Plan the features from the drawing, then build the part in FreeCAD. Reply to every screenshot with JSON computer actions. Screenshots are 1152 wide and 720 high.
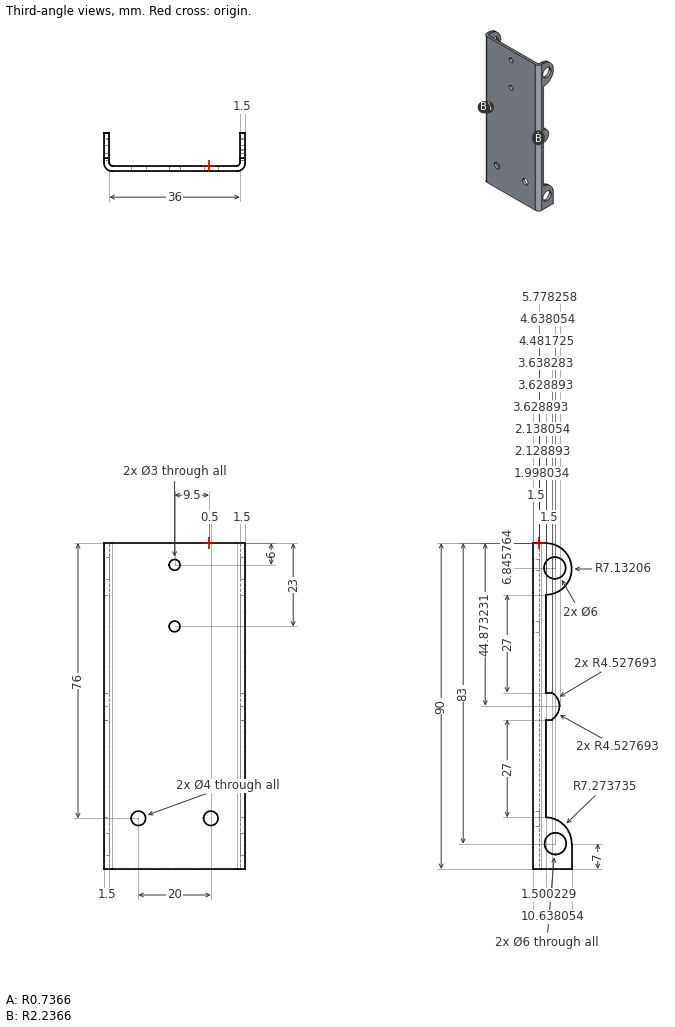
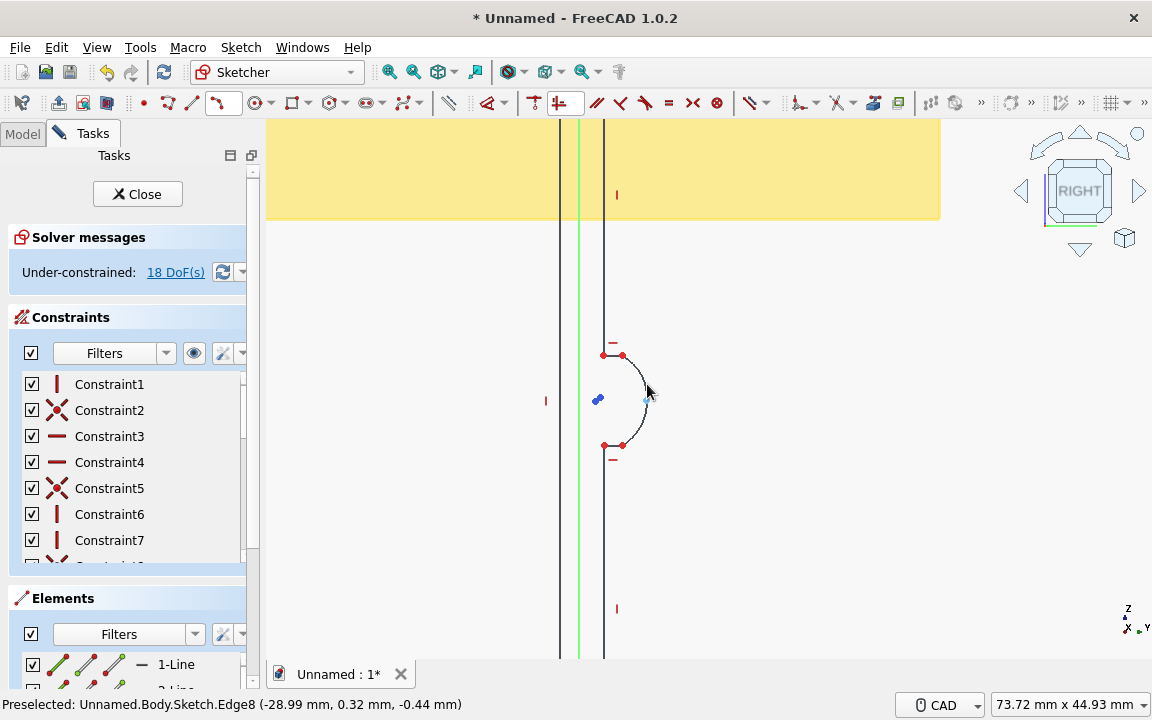
{"action": "left_click", "coordinate": [645, 384]}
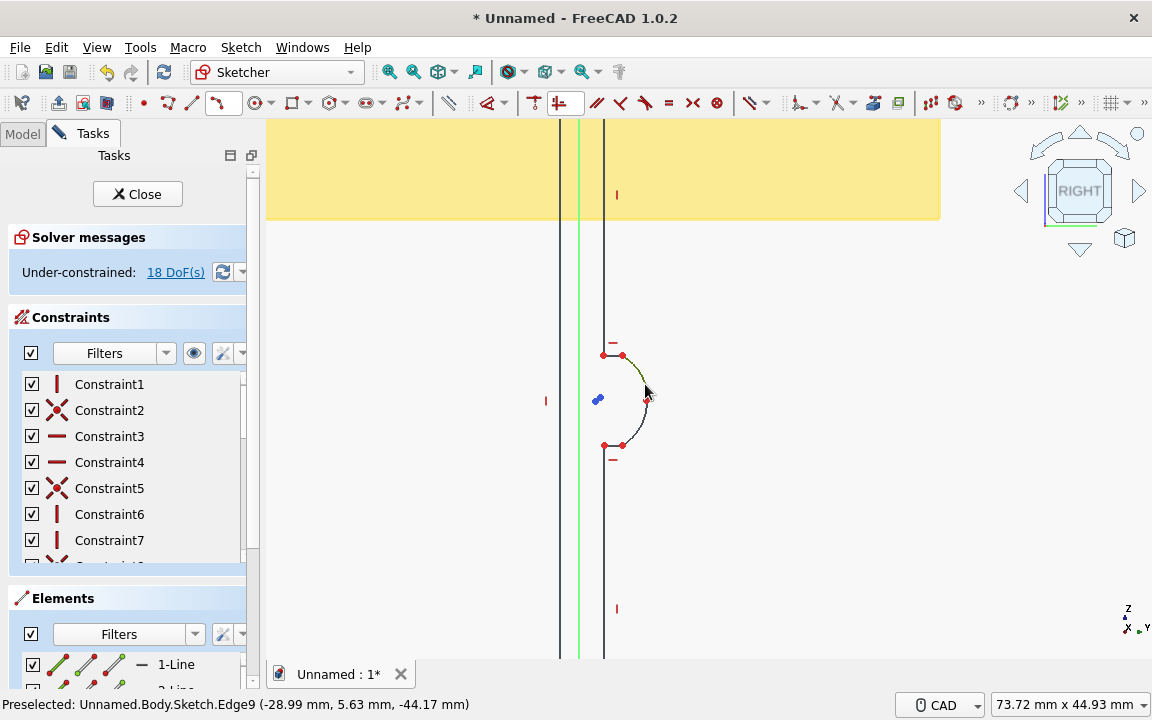
{"action": "left_click", "coordinate": [634, 435]}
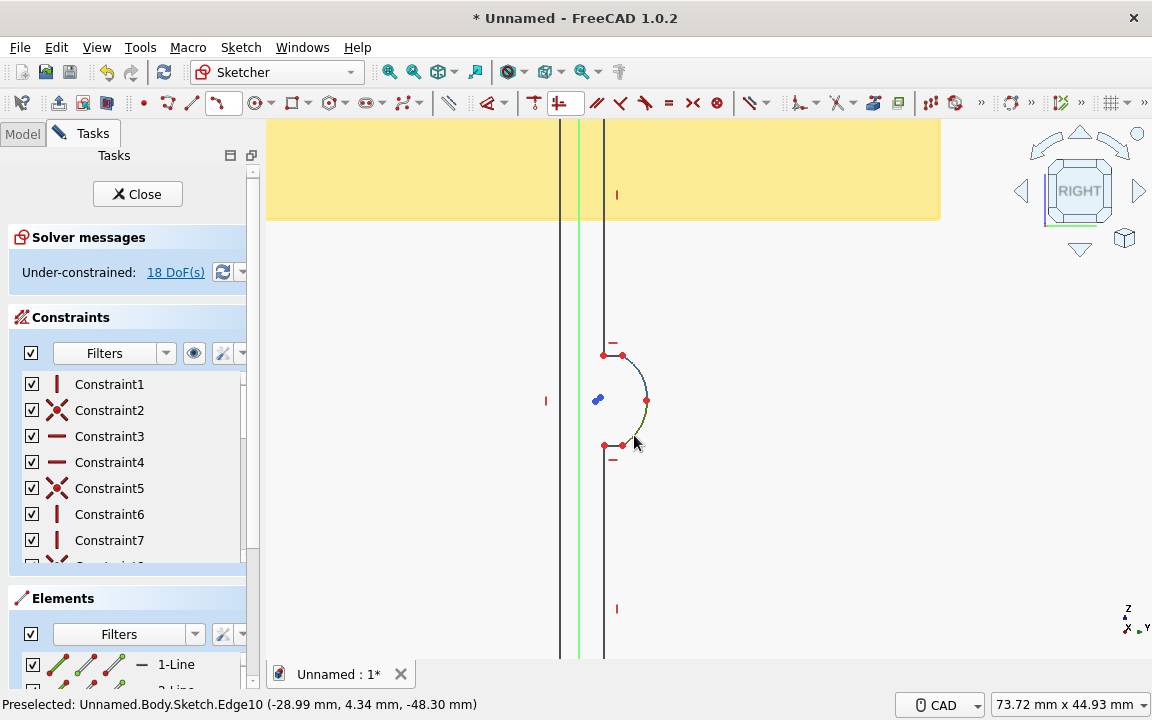
{"action": "key", "text": "e"}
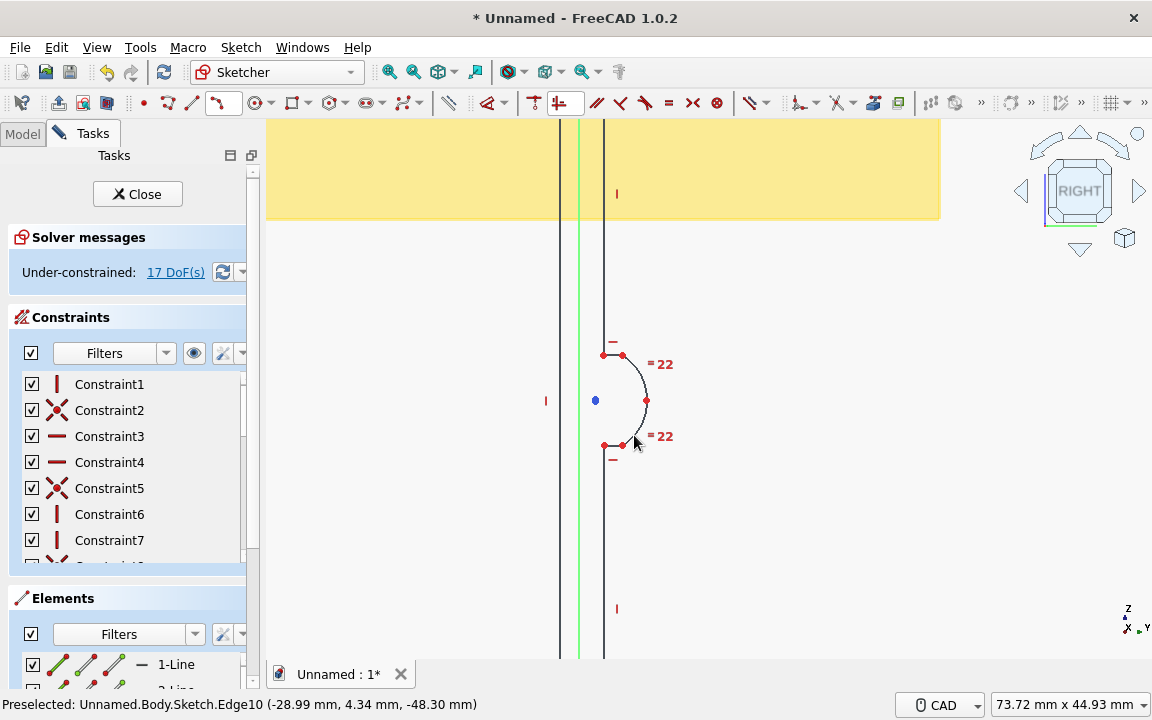
{"action": "left_click", "coordinate": [488, 104]}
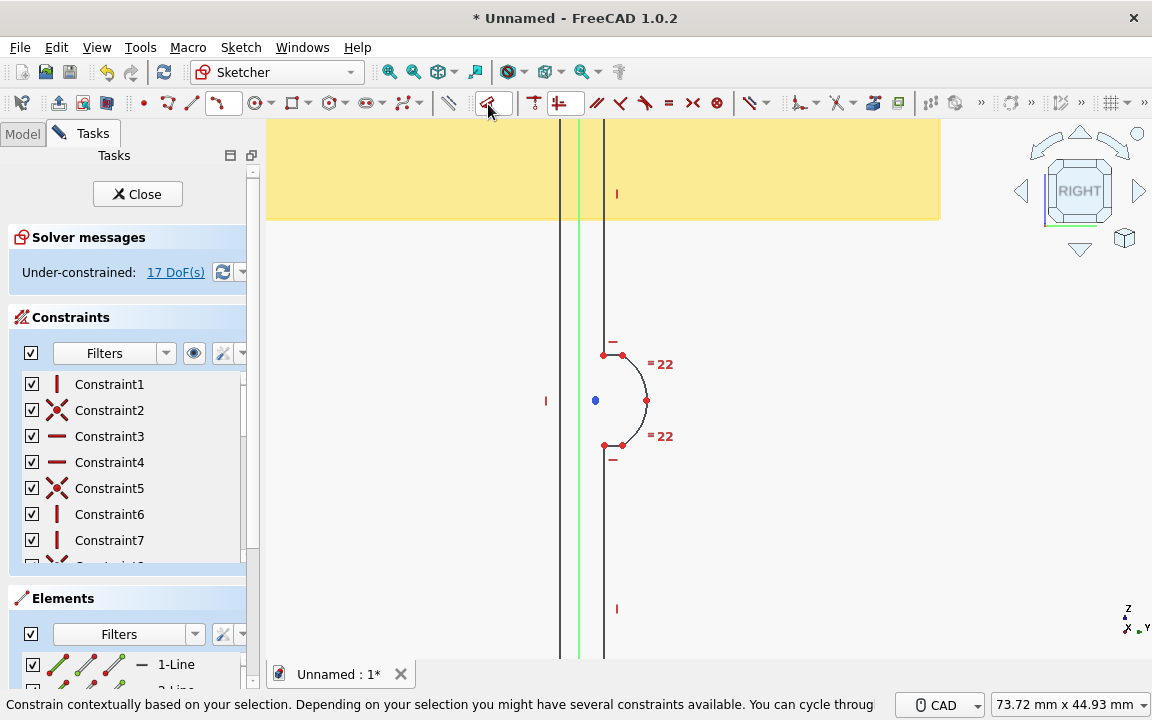
{"action": "left_click", "coordinate": [645, 385]}
{"action": "left_click", "coordinate": [676, 376]}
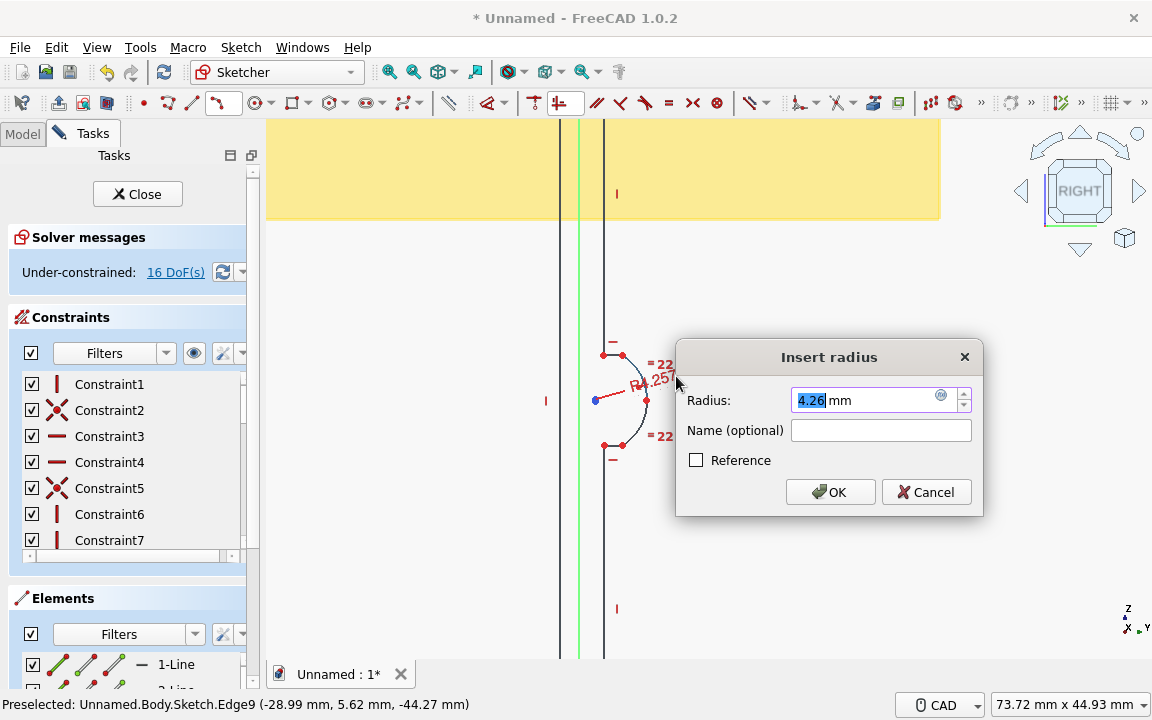
{"action": "type", "text": "4.527693"}
{"action": "key", "text": "Return"}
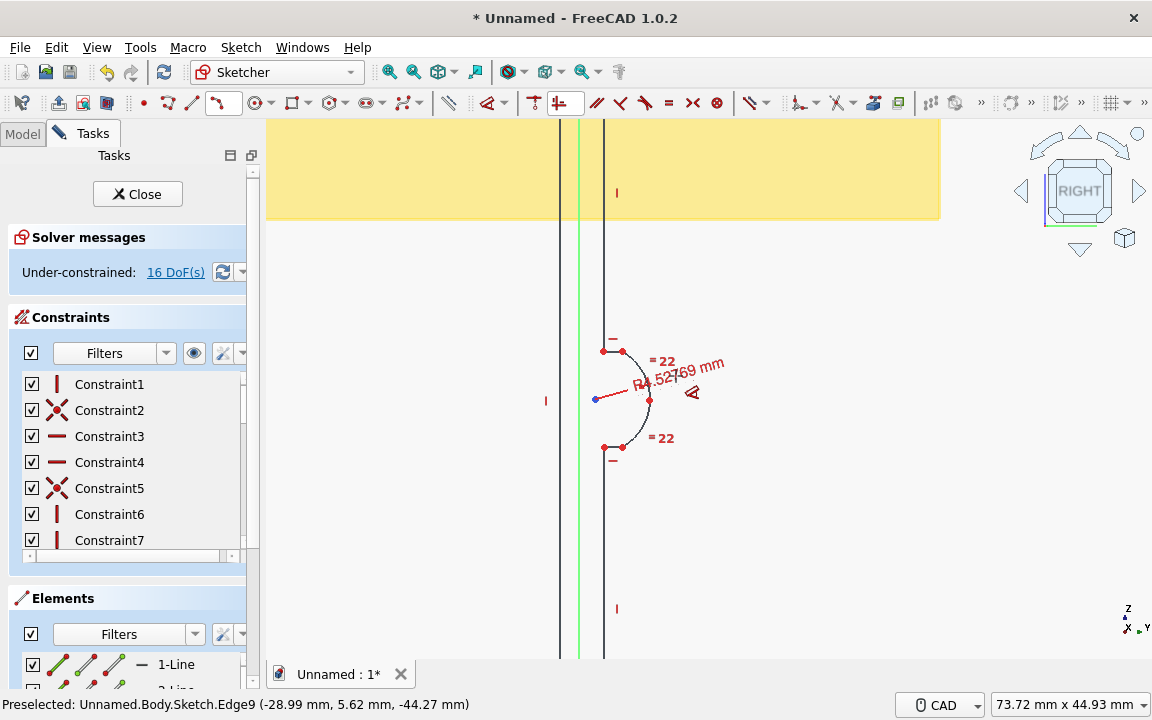
{"action": "scroll", "coordinate": [647, 384], "scroll_direction": "down", "scroll_amount": 6}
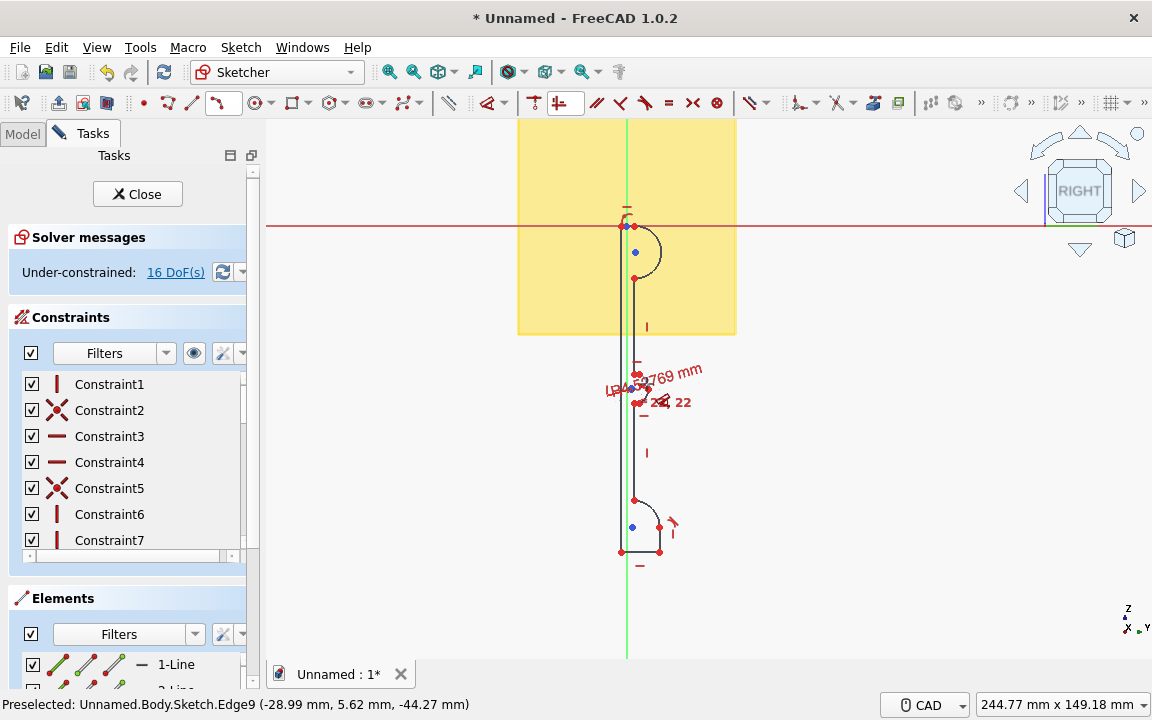
{"action": "scroll", "coordinate": [657, 516], "scroll_direction": "up", "scroll_amount": 3}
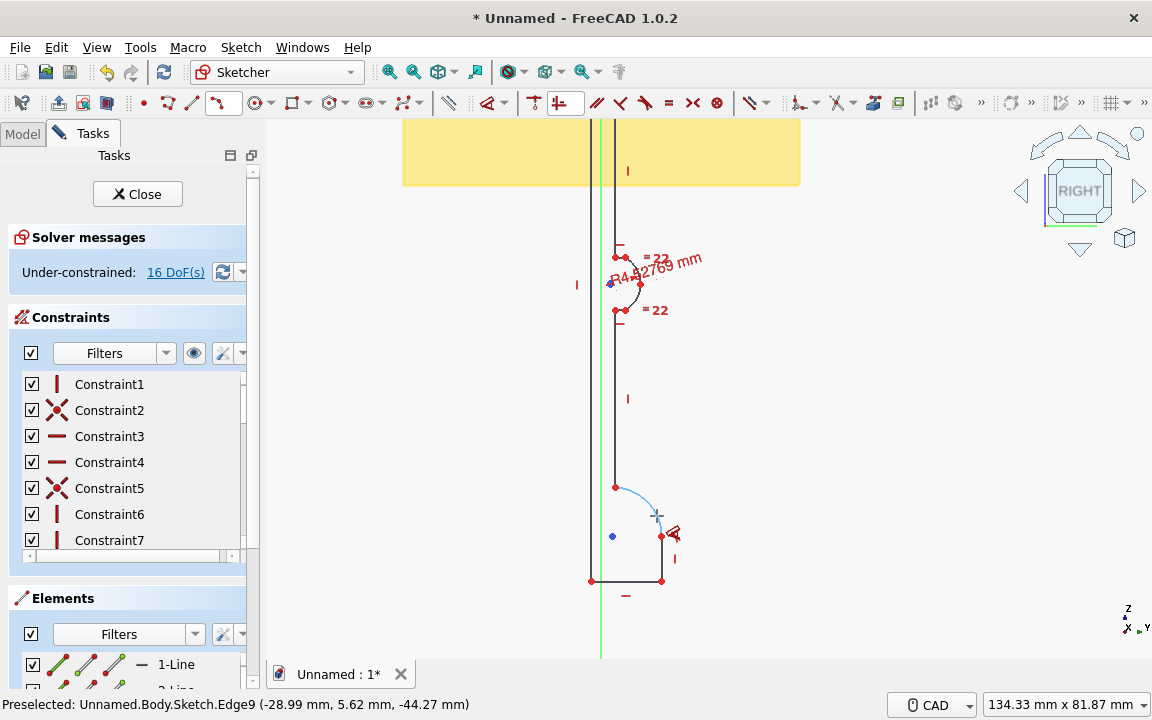
{"action": "left_click", "coordinate": [657, 515]}
{"action": "left_click", "coordinate": [686, 501]}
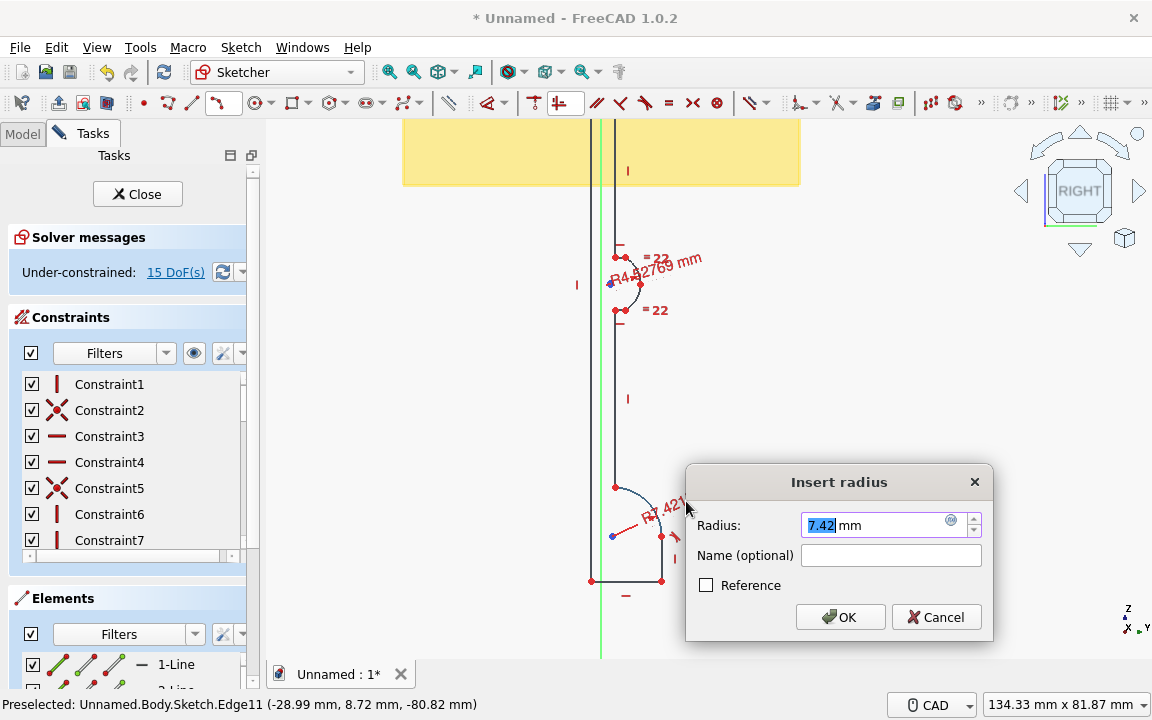
{"action": "type", "text": "7.273735"}
{"action": "key", "text": "Return"}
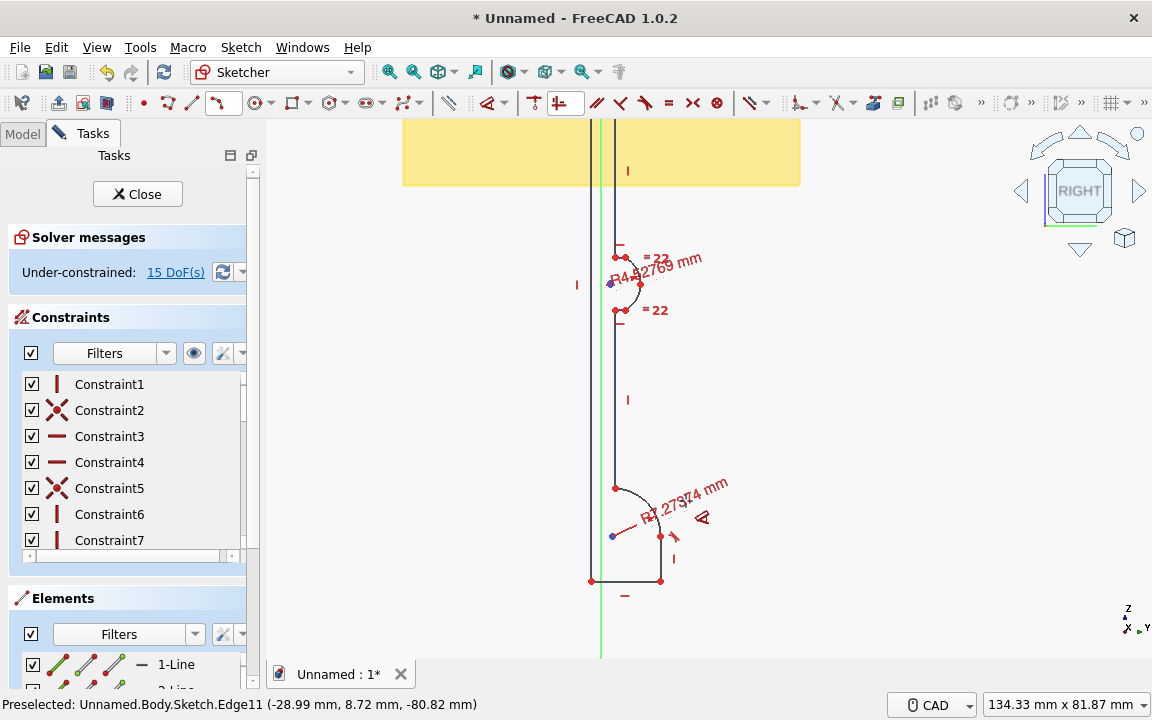
{"action": "scroll", "coordinate": [657, 517], "scroll_direction": "down", "scroll_amount": 3}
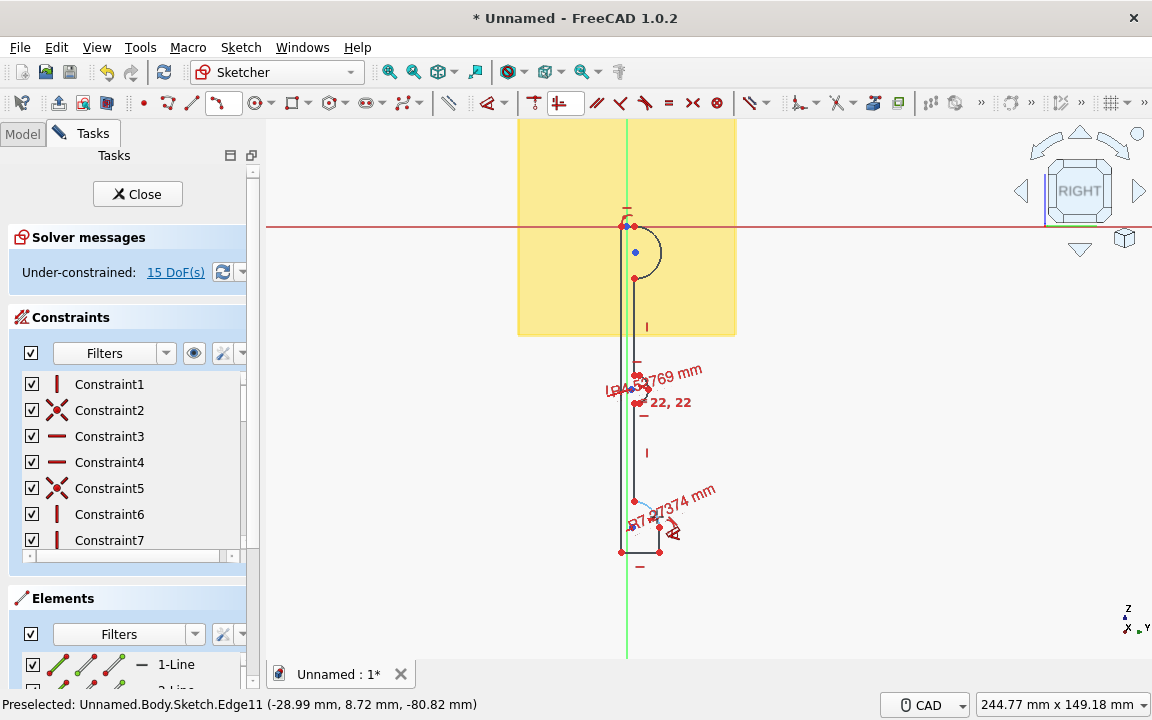
{"action": "scroll", "coordinate": [656, 268], "scroll_direction": "up", "scroll_amount": 3}